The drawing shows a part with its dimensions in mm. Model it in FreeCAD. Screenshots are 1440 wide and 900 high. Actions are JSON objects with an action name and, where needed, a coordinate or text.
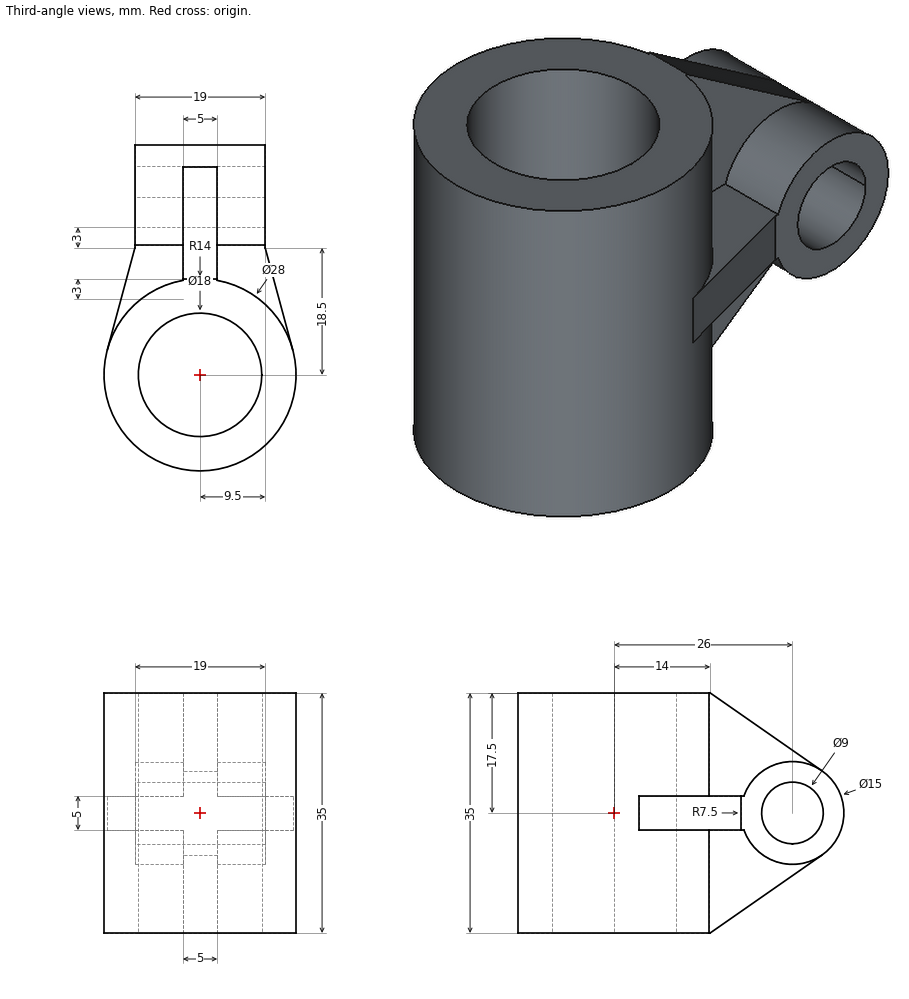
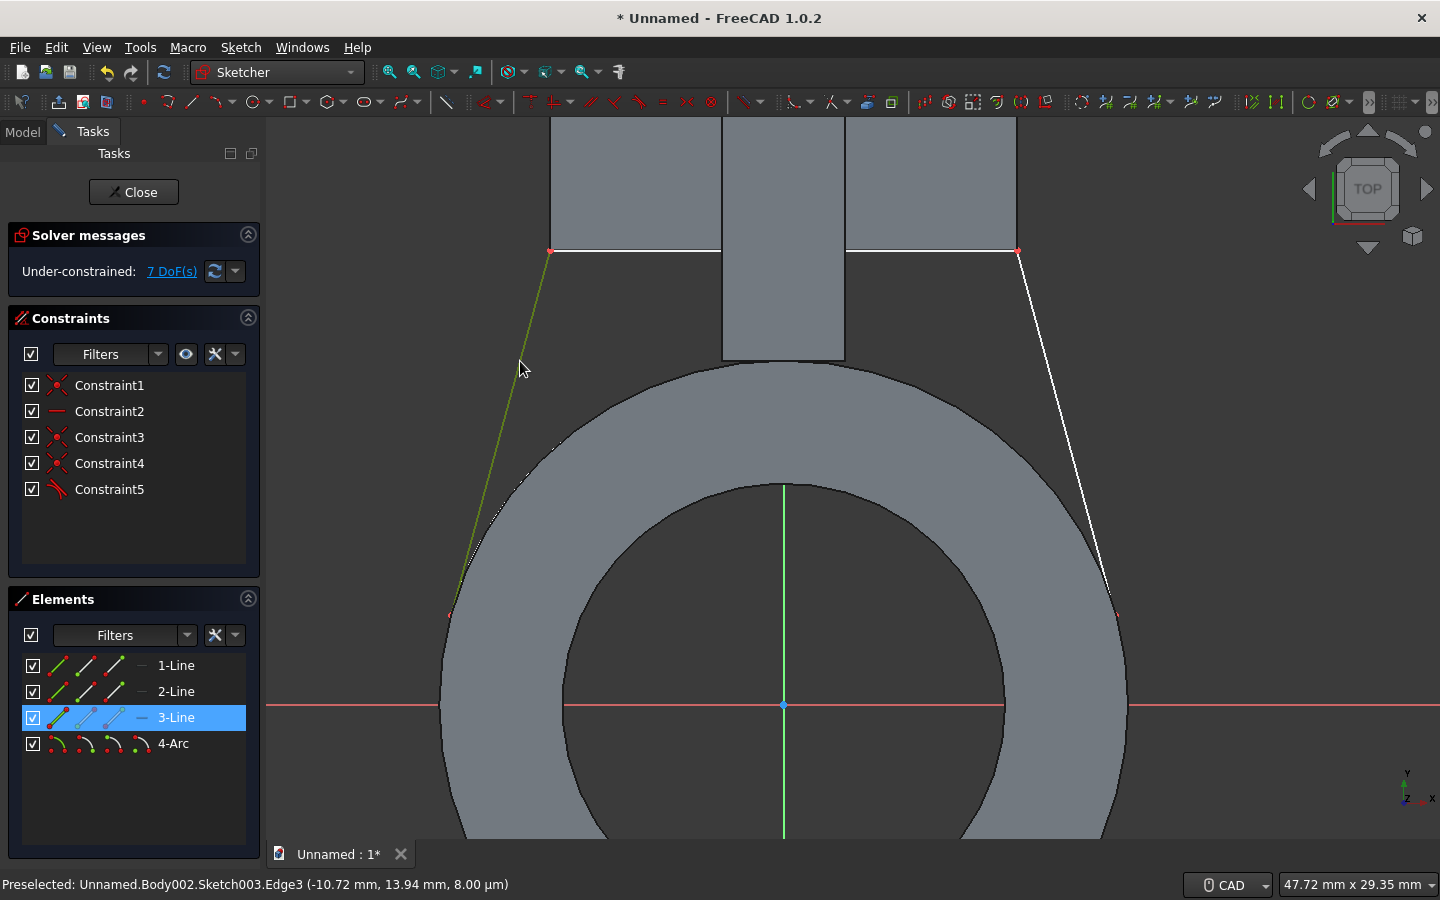
{"action": "left_click", "coordinate": [955, 407]}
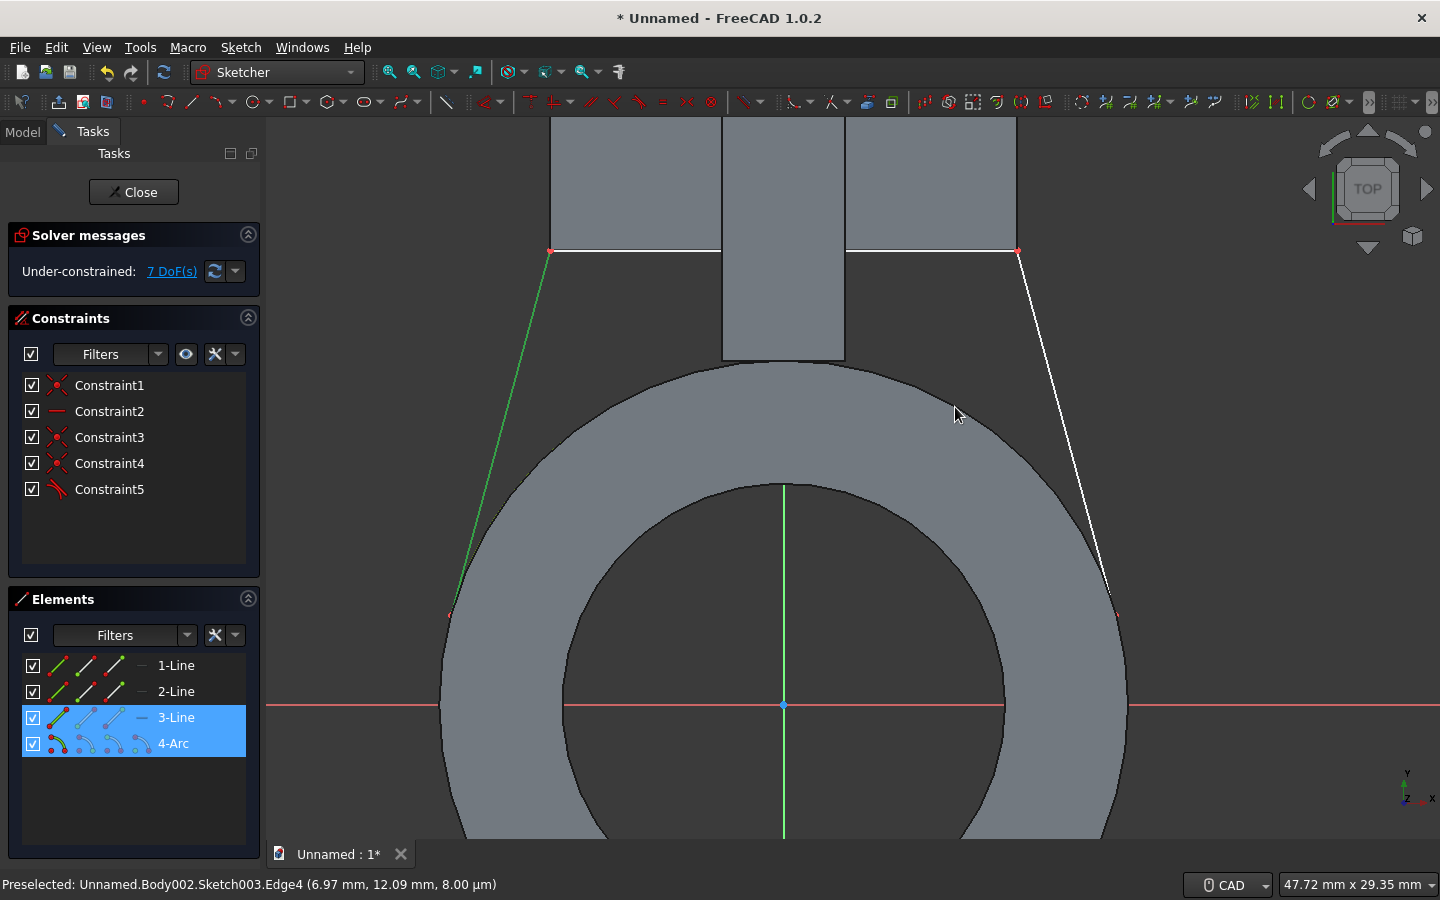
{"action": "key", "text": "t"}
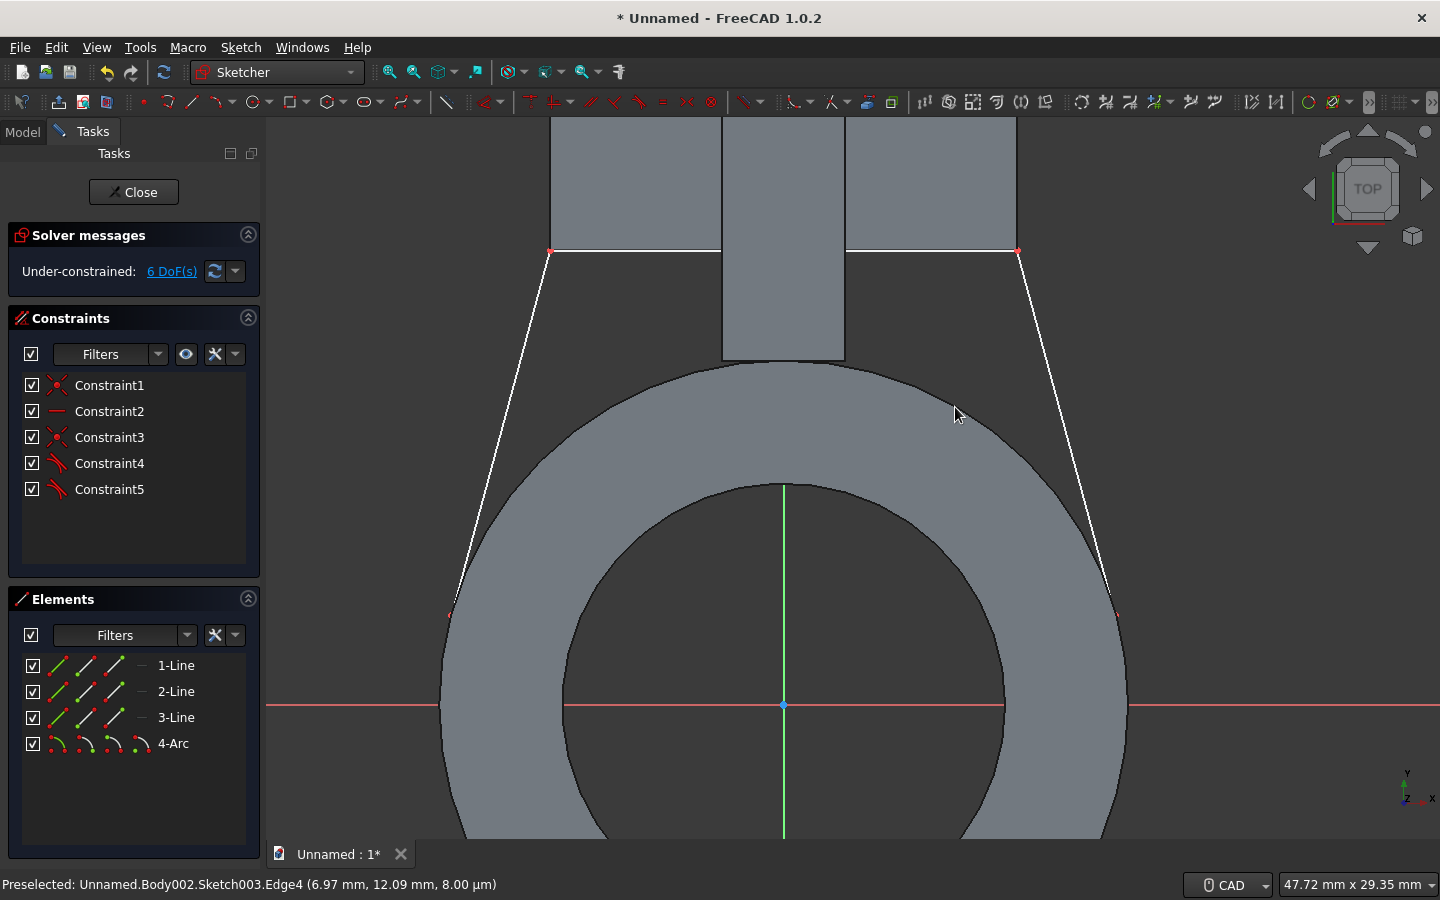
{"action": "left_click_drag", "start_coordinate": [774, 695], "coordinate": [794, 716]}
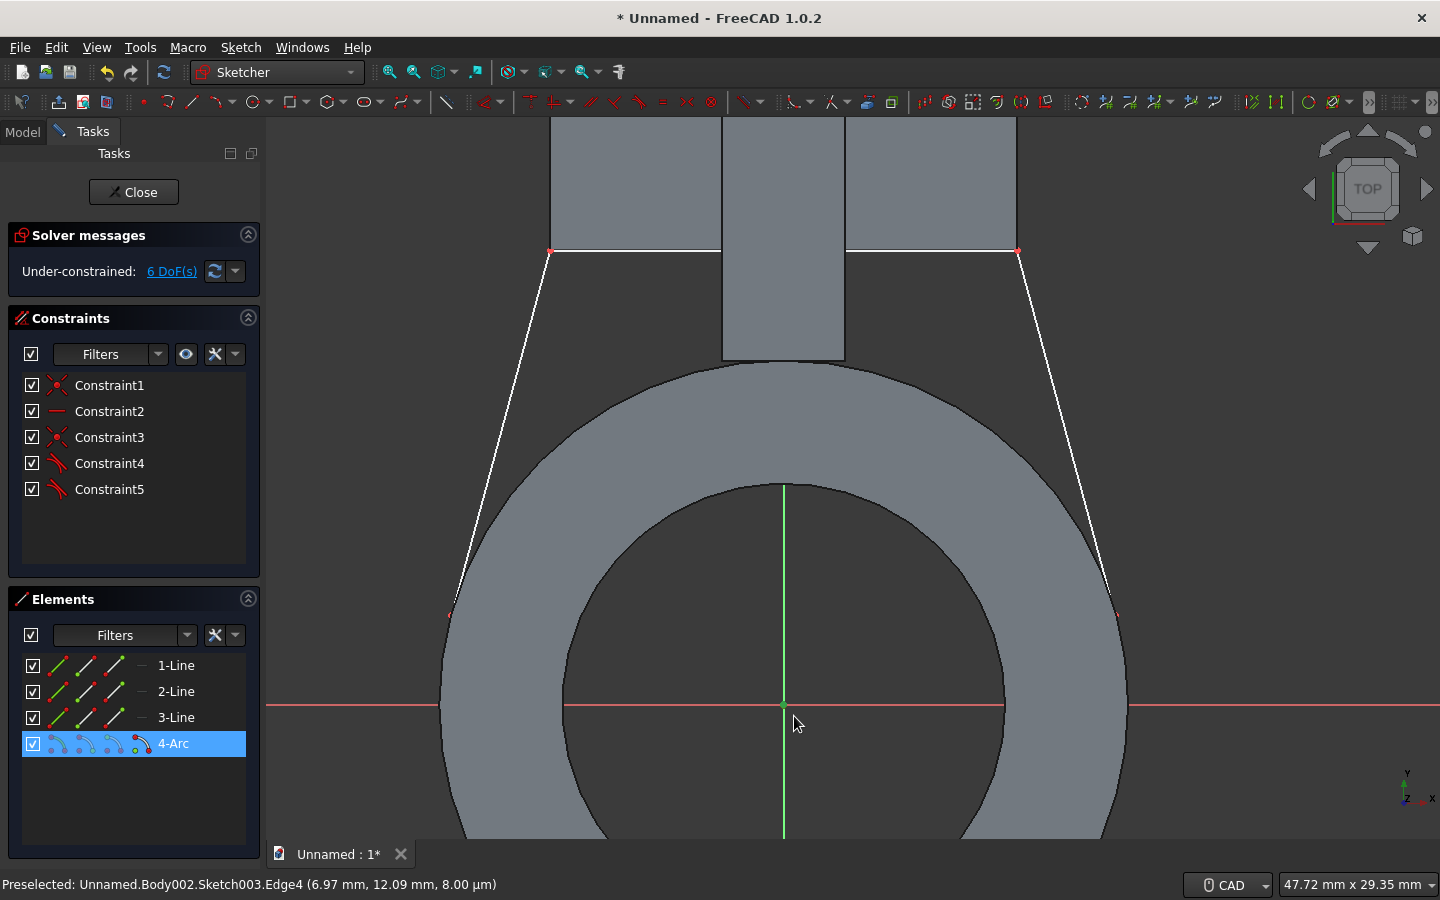
{"action": "key", "text": "c"}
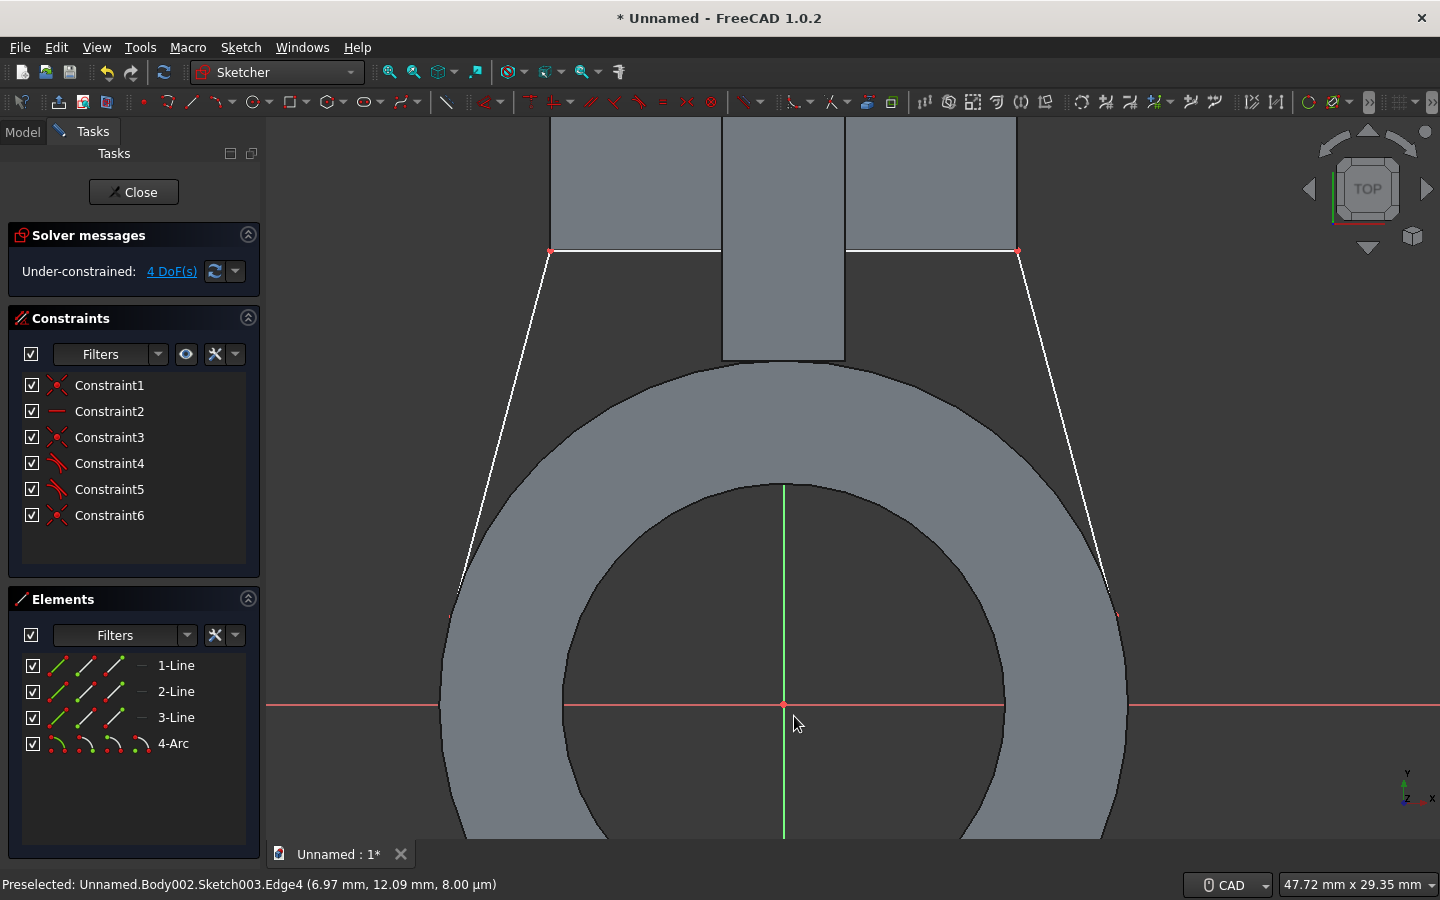
{"action": "left_click", "coordinate": [484, 102]}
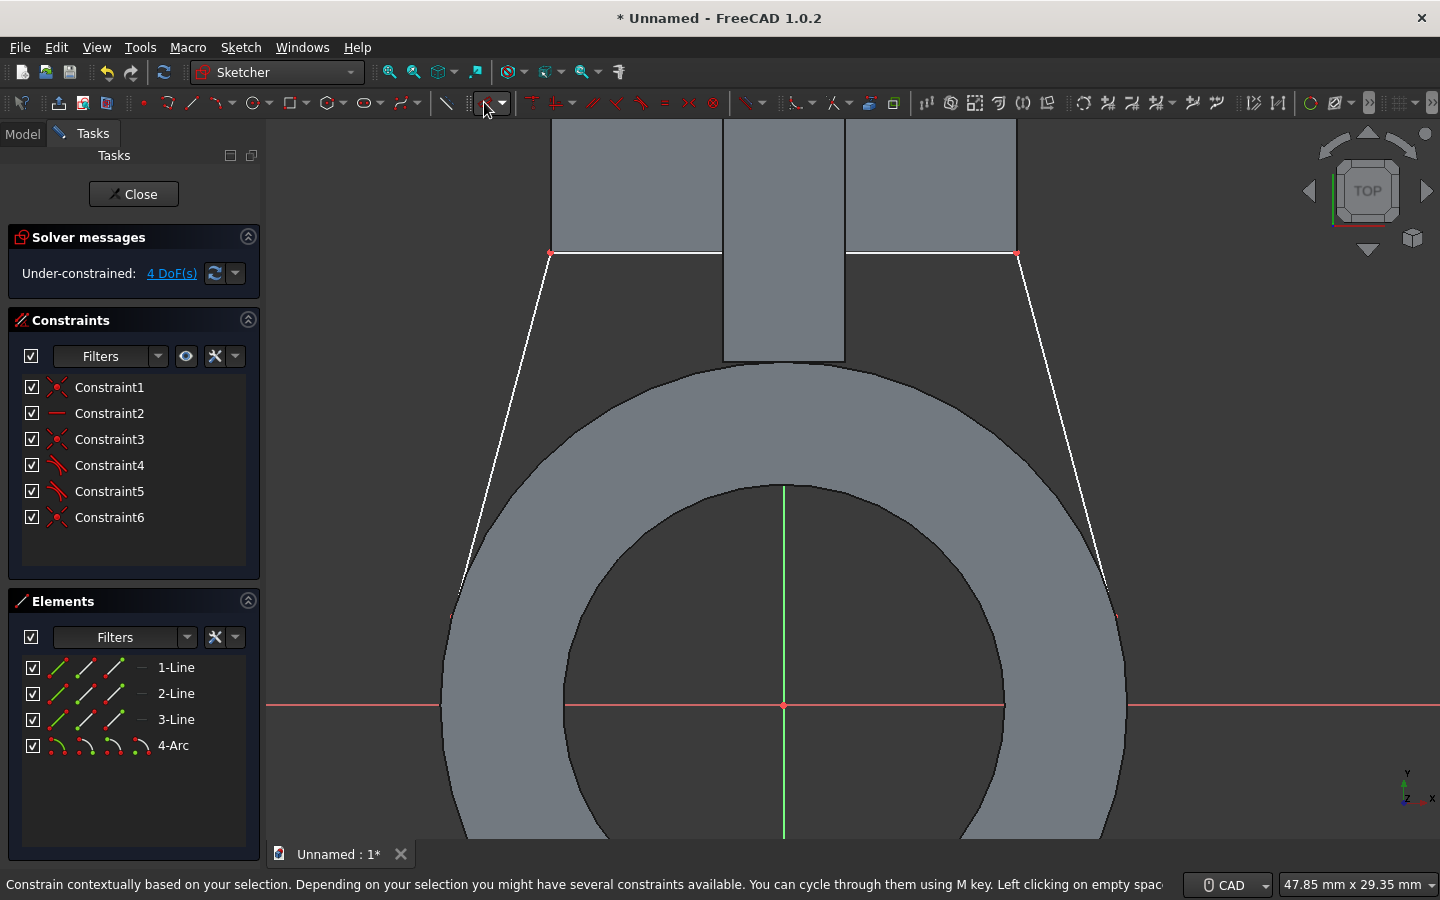
{"action": "left_click", "coordinate": [955, 409]}
{"action": "left_click", "coordinate": [971, 381]}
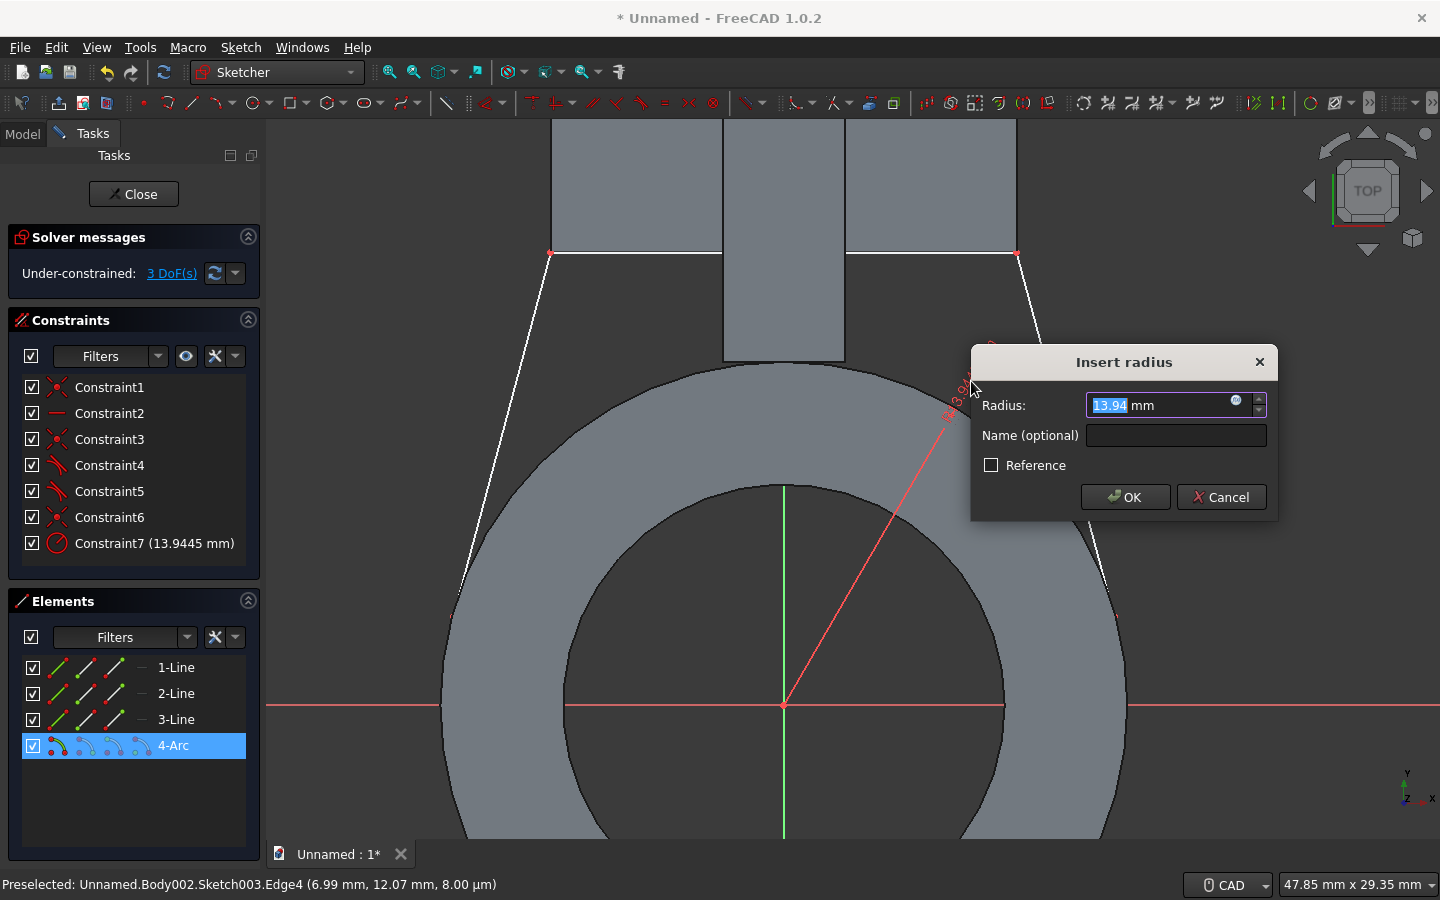
{"action": "type", "text": "14"}
{"action": "key", "text": "Return"}